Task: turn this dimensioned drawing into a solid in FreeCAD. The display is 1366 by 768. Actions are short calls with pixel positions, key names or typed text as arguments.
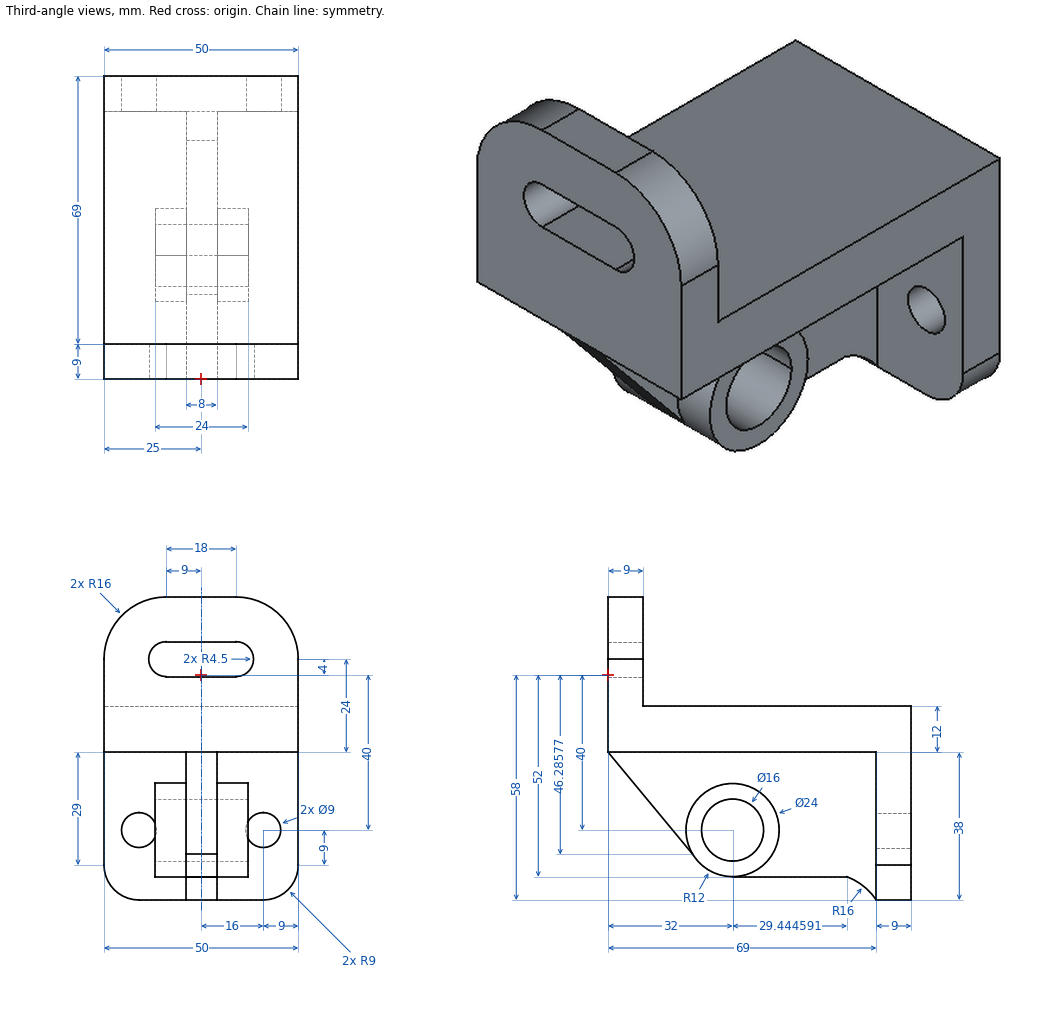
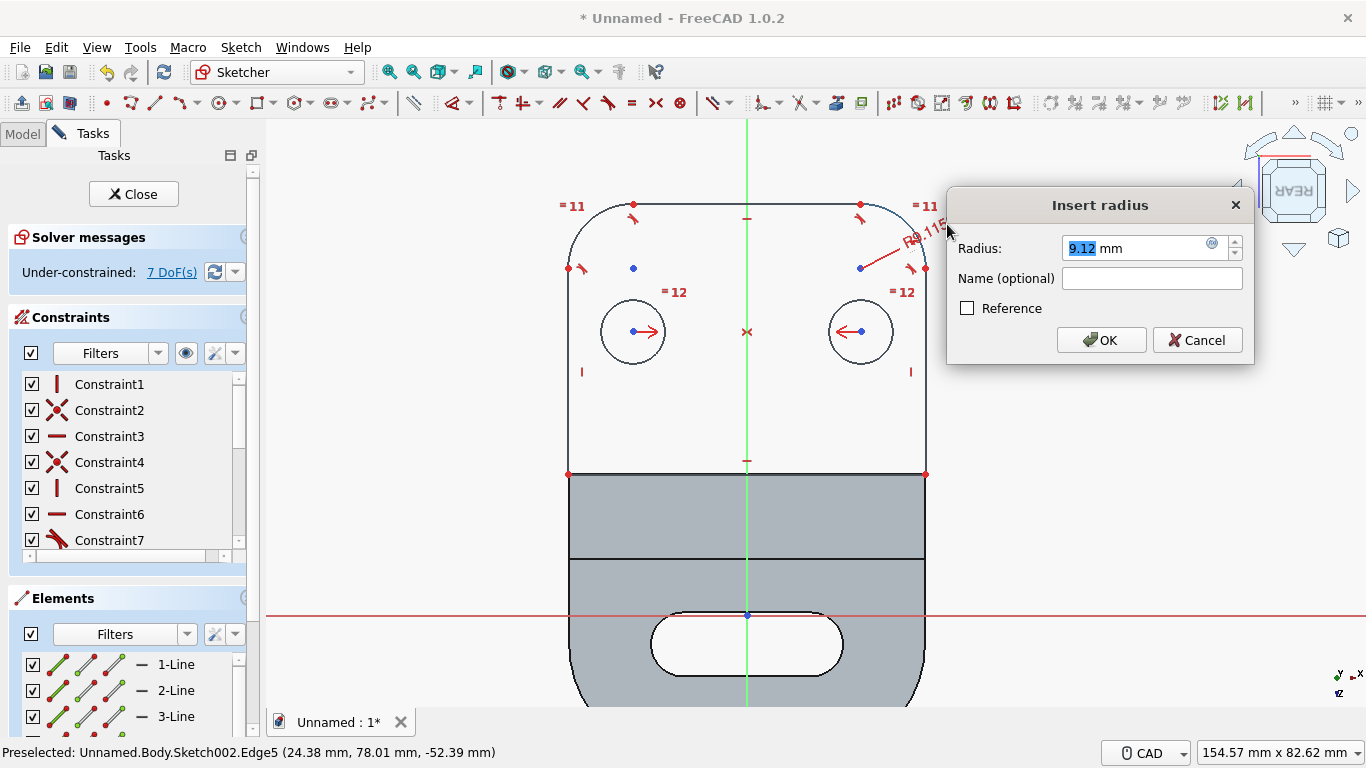
text(9)
key(Return)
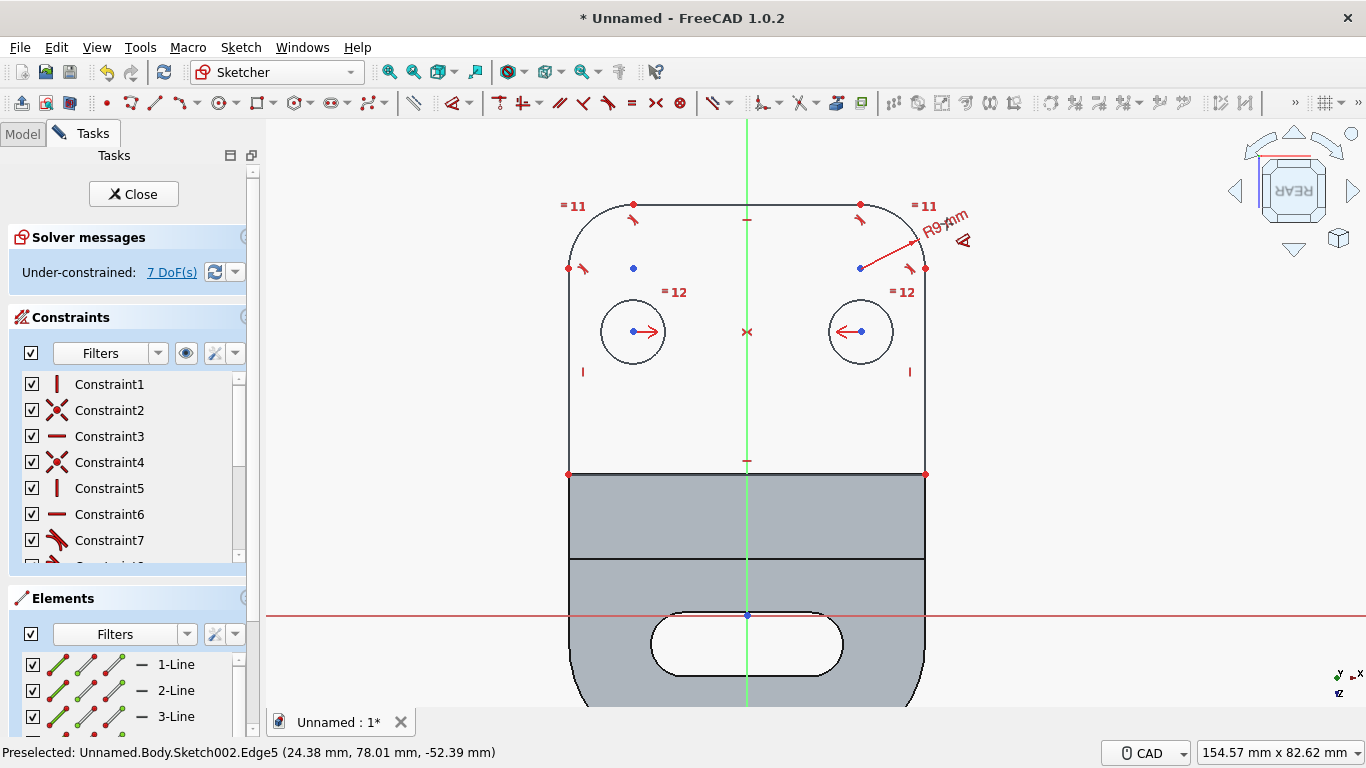
click(883, 309)
click(905, 286)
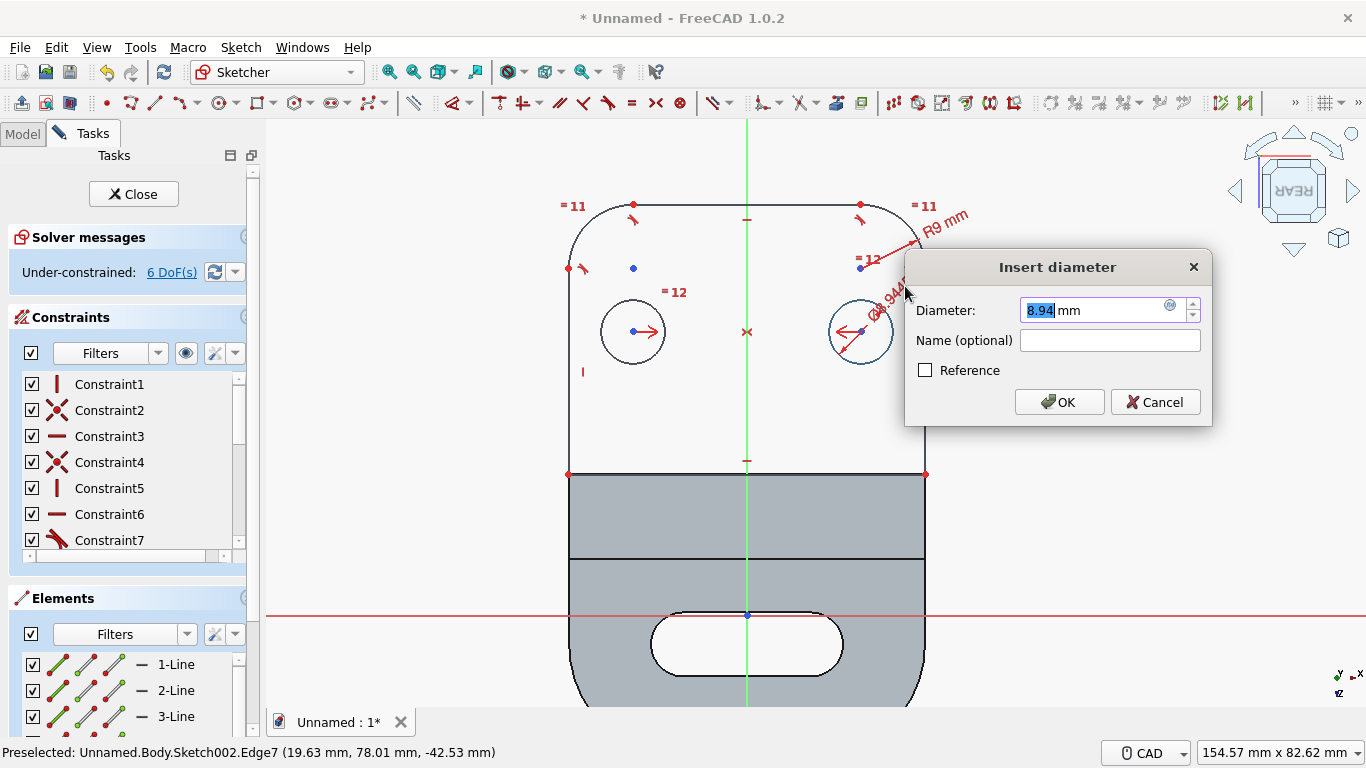
text(9)
key(Return)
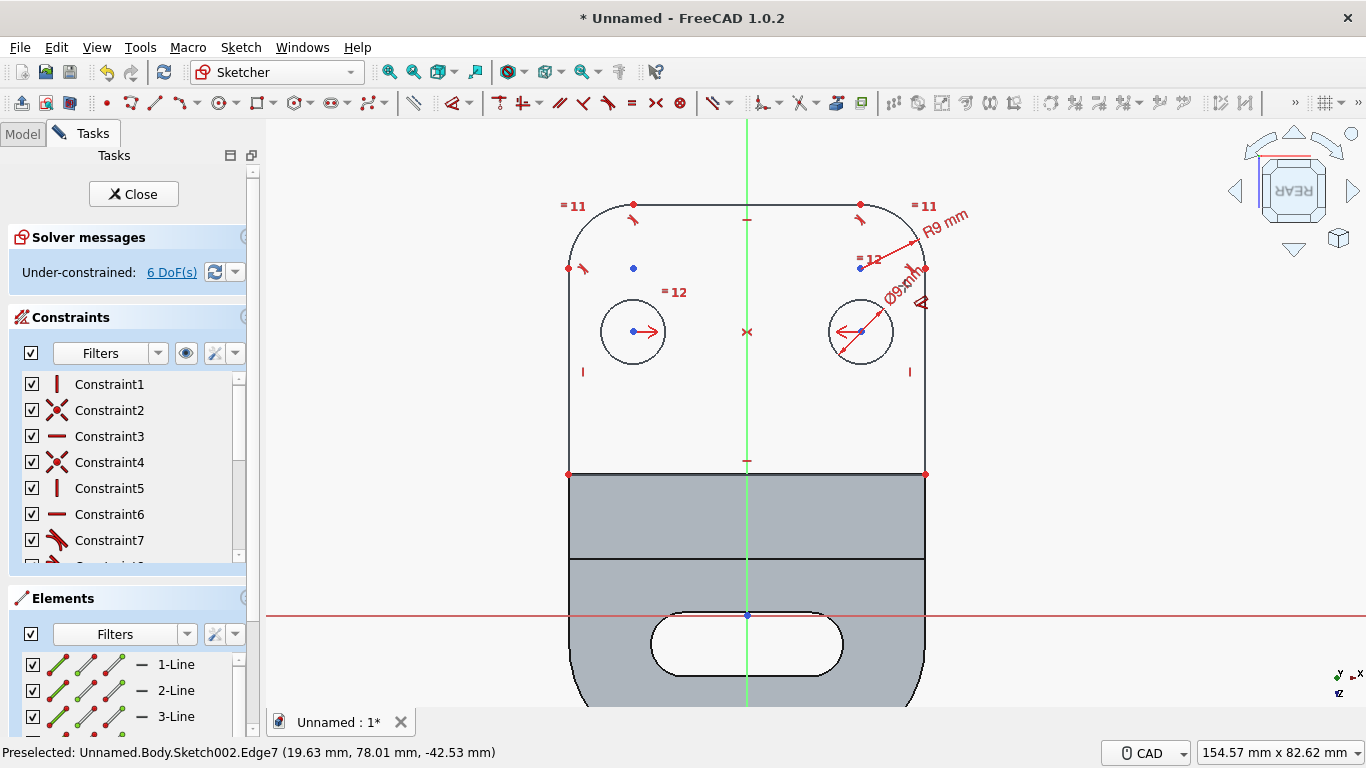
click(569, 331)
click(535, 372)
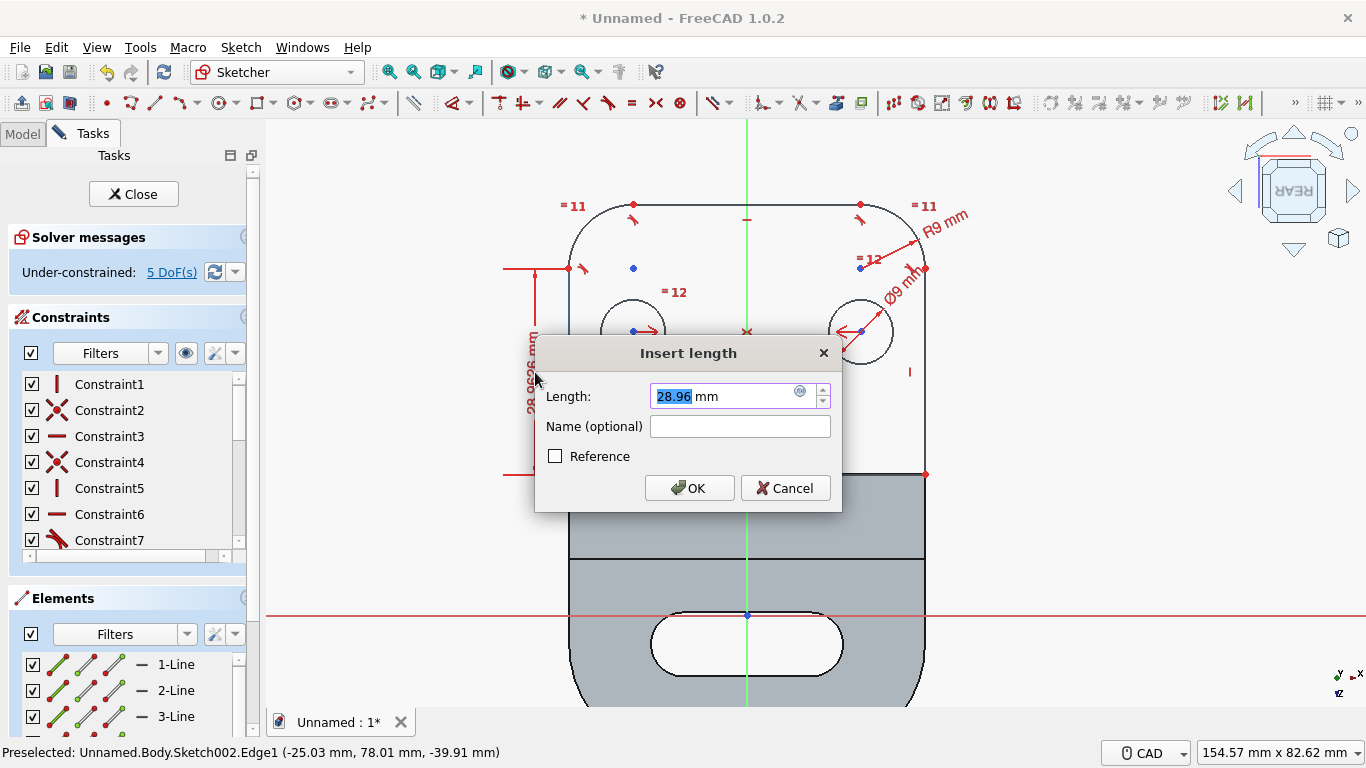
text(29)
key(Return)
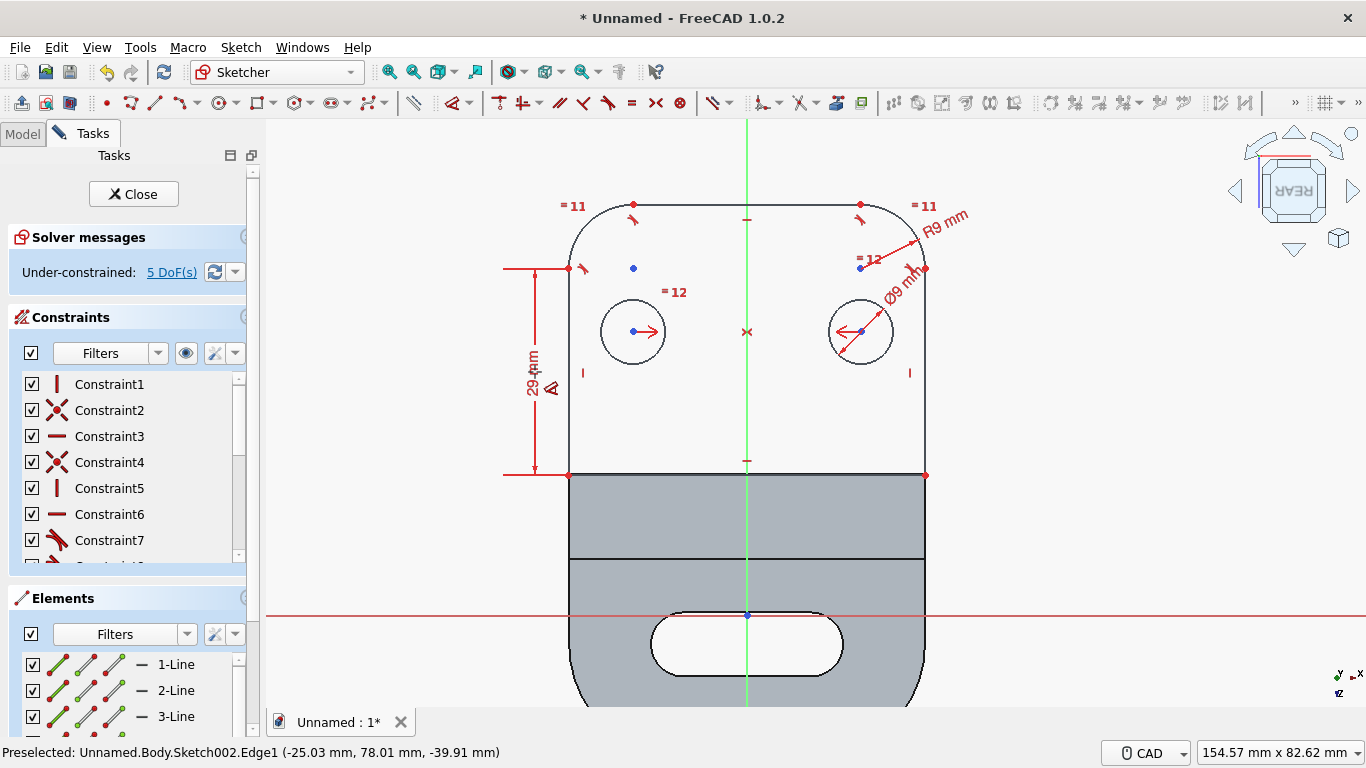
click(676, 475)
click(665, 509)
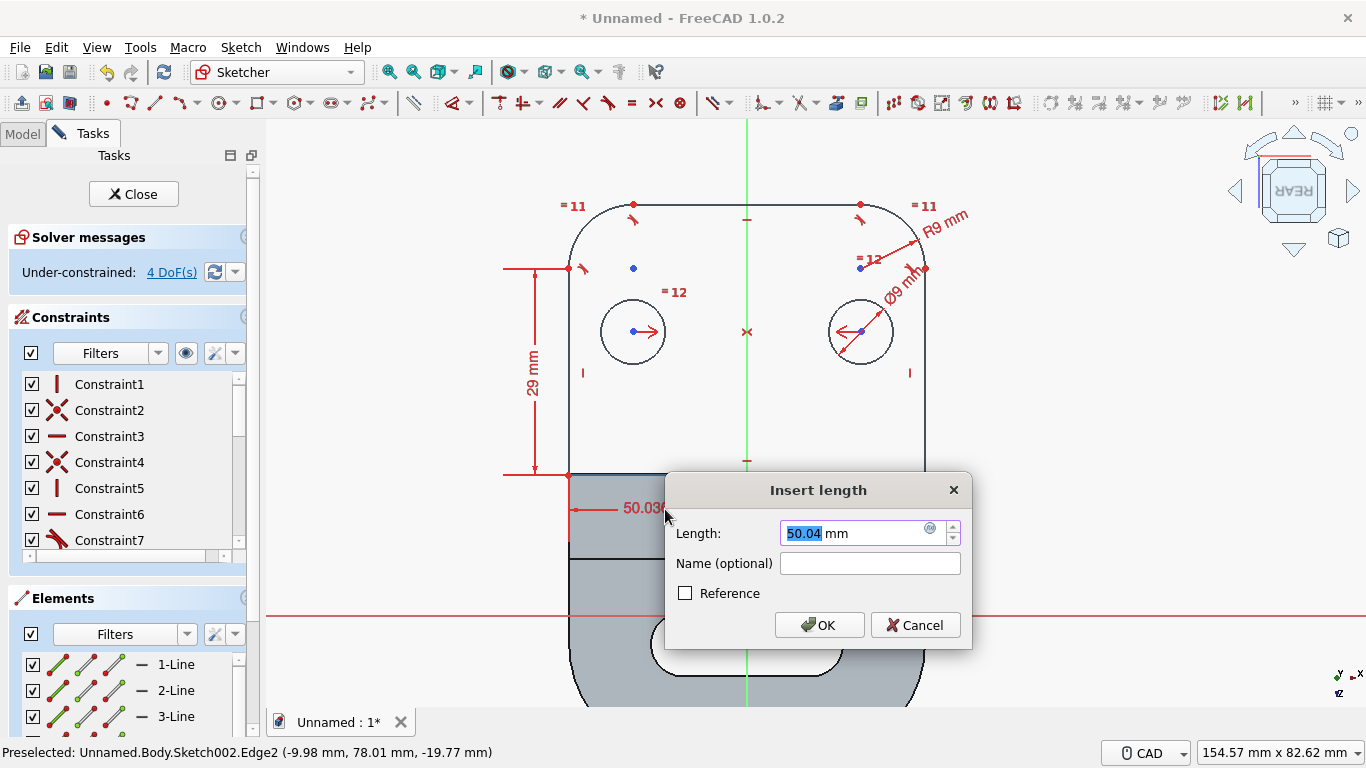
text(50)
key(Return)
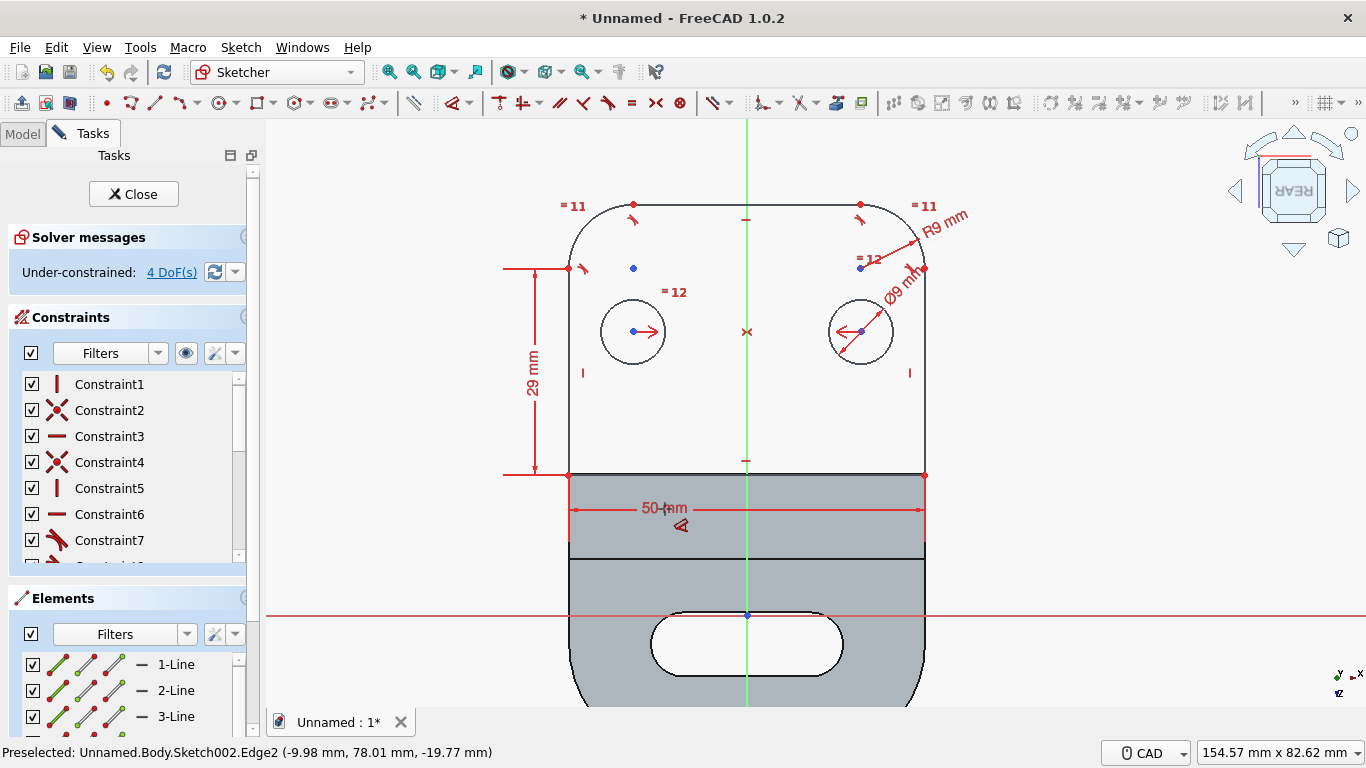
click(861, 332)
click(804, 650)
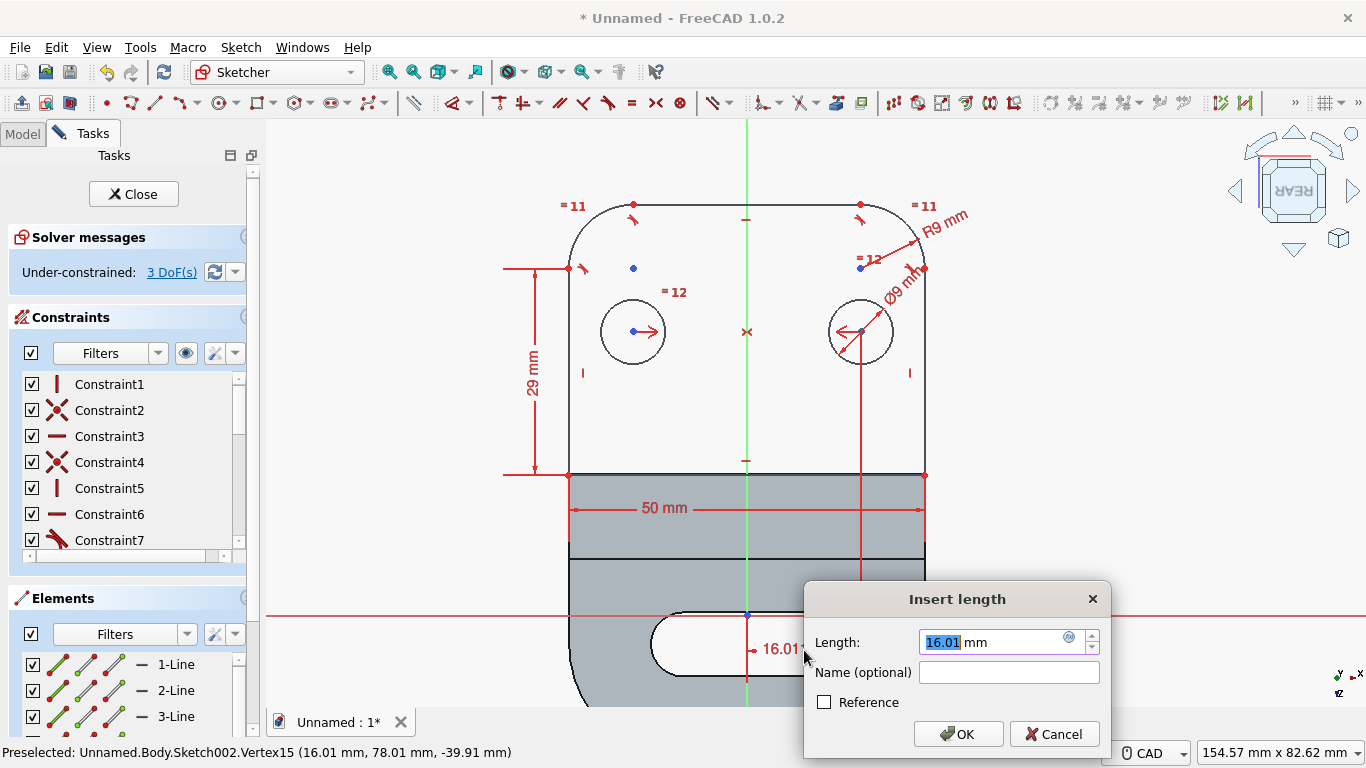
text(16)
key(Return)